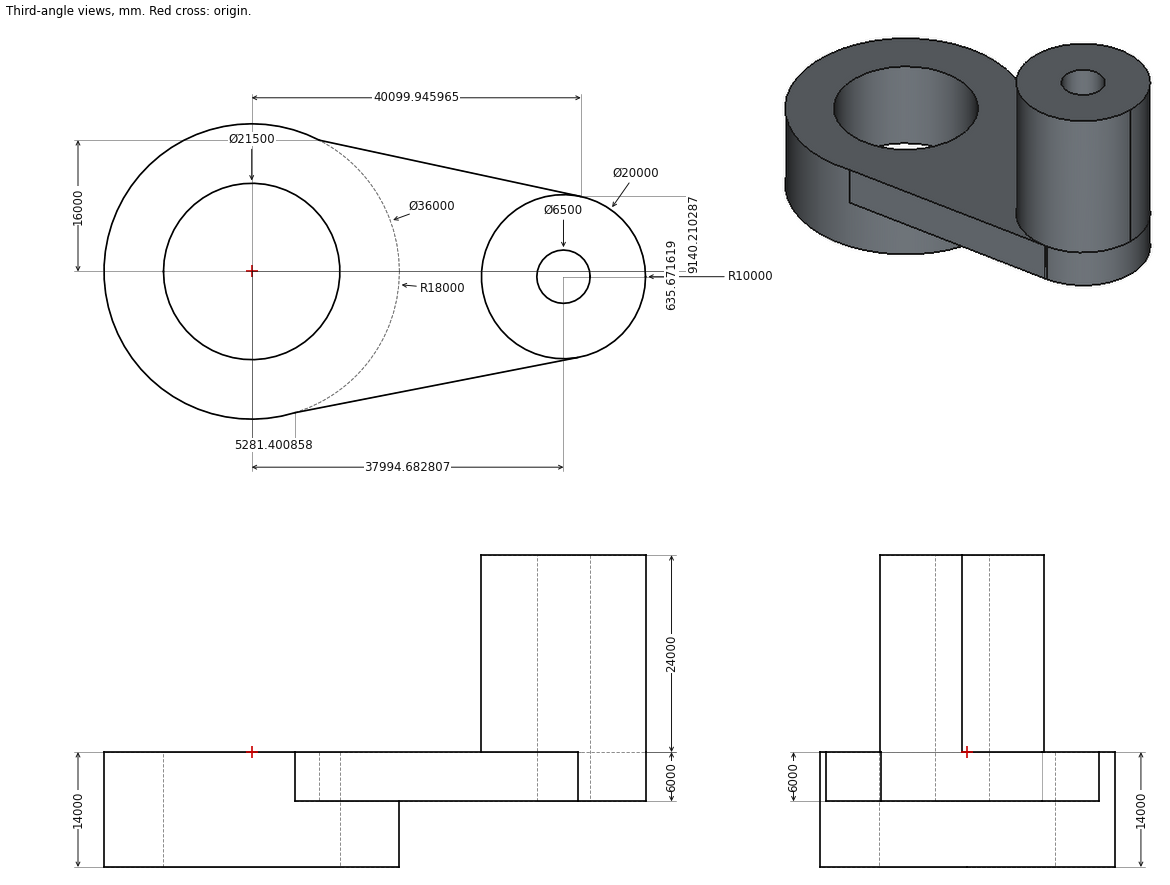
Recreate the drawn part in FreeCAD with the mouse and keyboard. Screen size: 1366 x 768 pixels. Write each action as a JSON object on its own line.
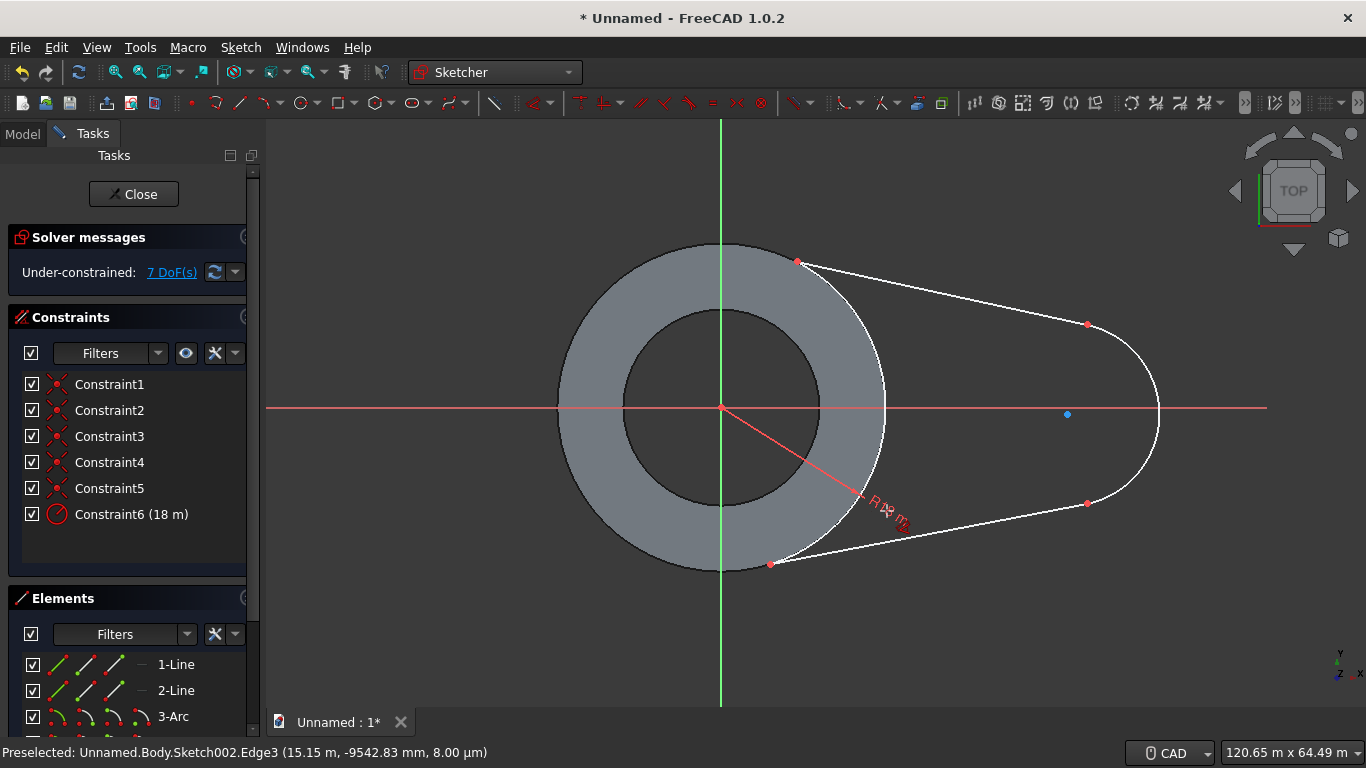
{"action": "left_click", "coordinate": [1146, 462]}
{"action": "left_click", "coordinate": [1173, 479]}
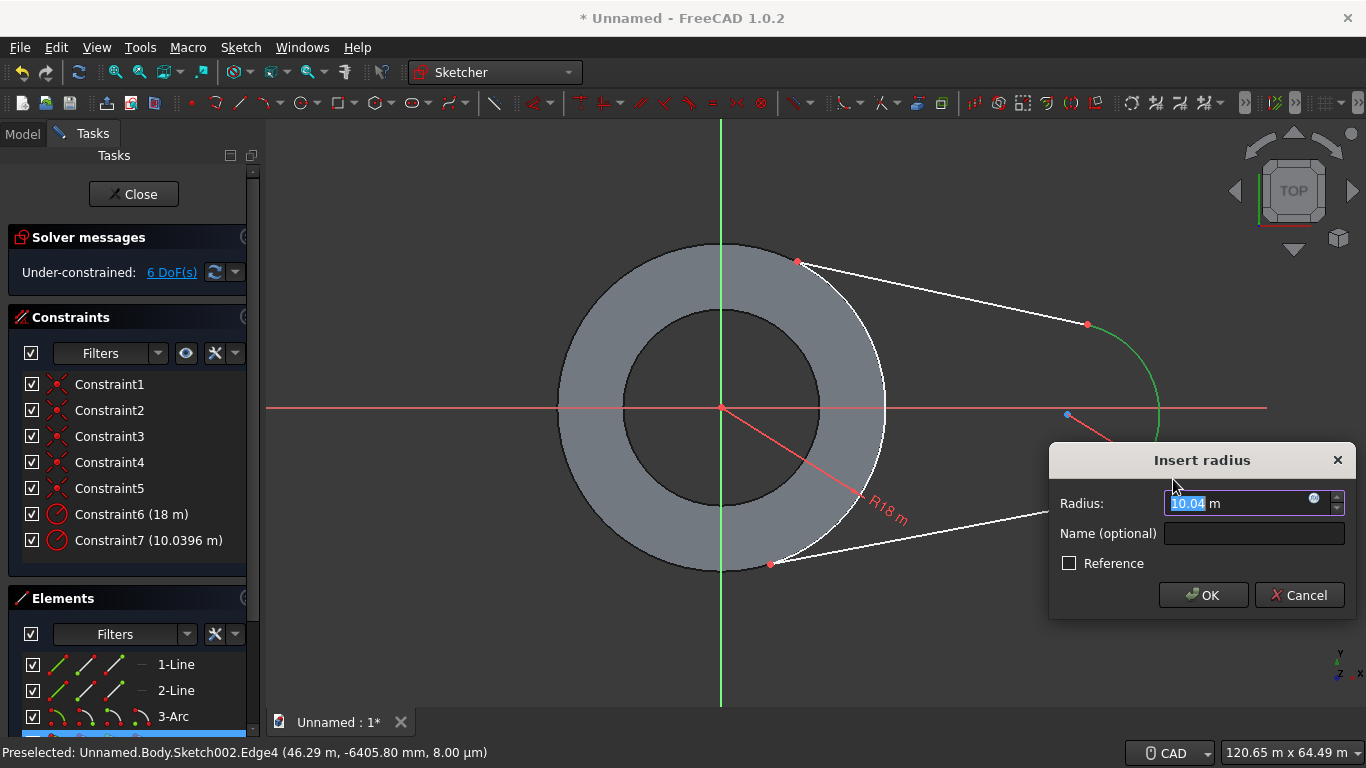
{"action": "key", "text": "ctrl+a"}
{"action": "type", "text": "10000 mm"}
{"action": "key", "text": "Return"}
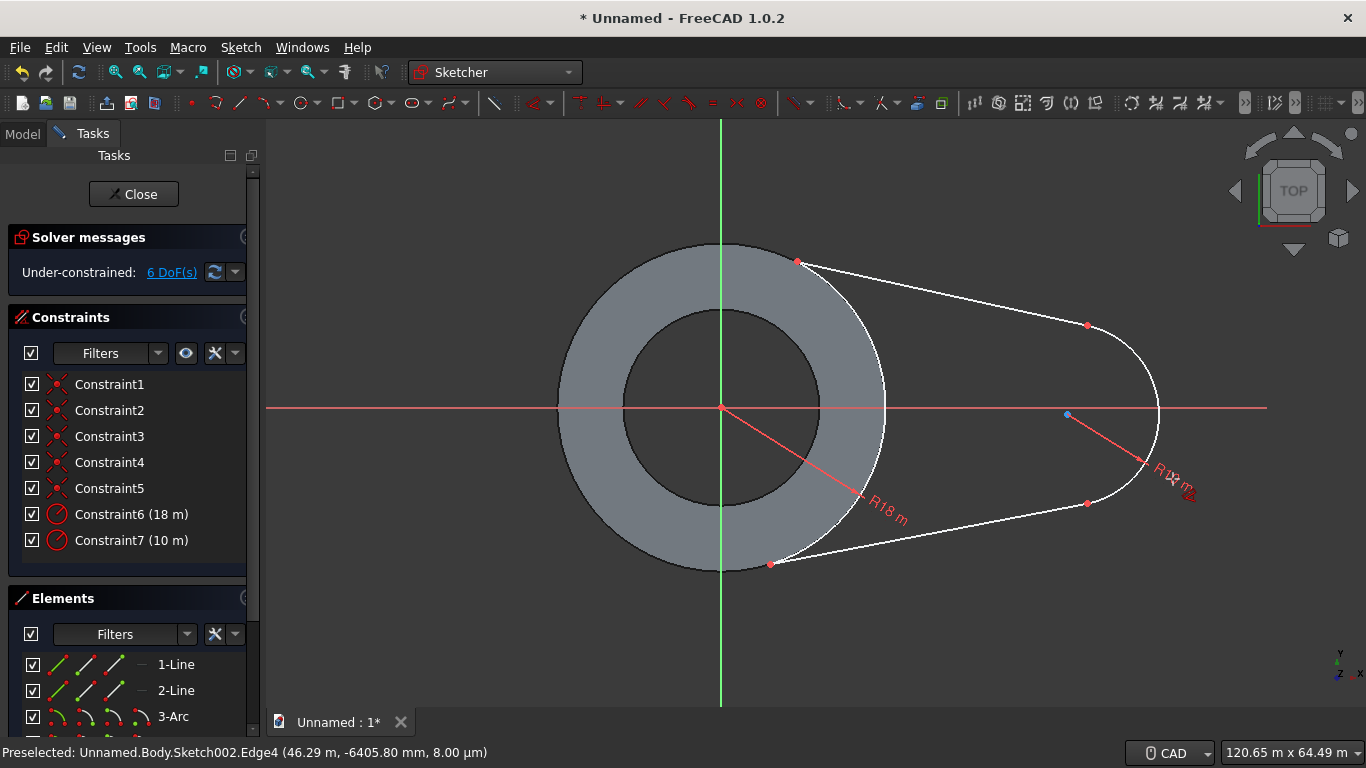
{"action": "left_click", "coordinate": [797, 262]}
{"action": "left_click", "coordinate": [687, 335]}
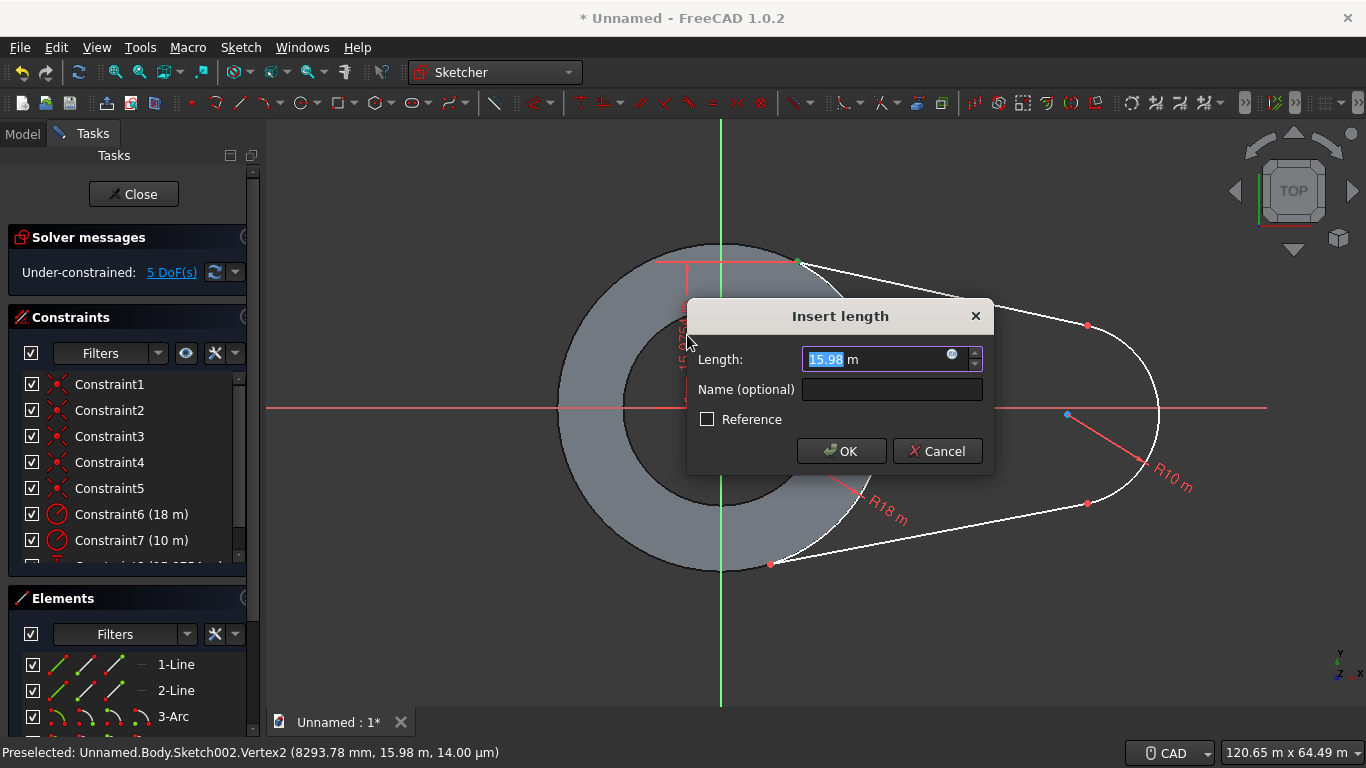
{"action": "key", "text": "ctrl+a"}
{"action": "type", "text": "16000 mm"}
{"action": "key", "text": "Return"}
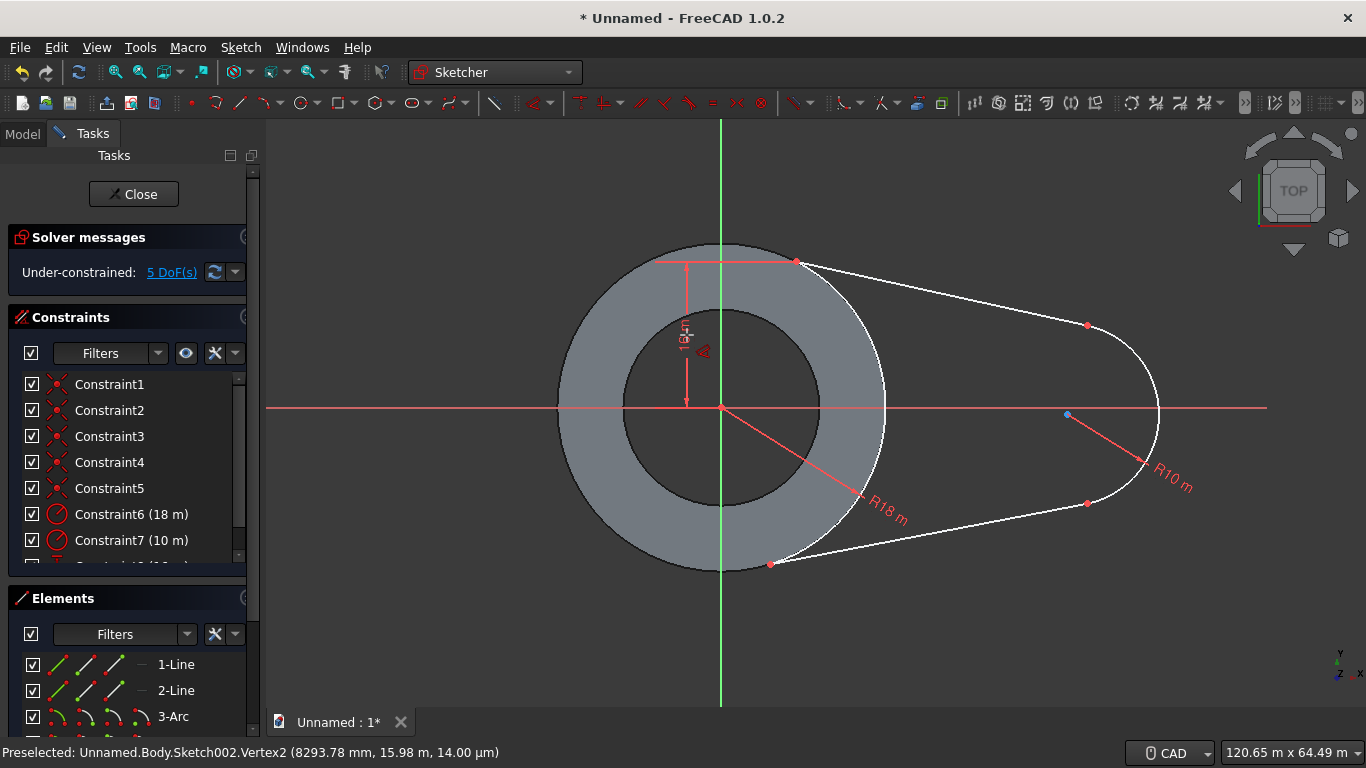
{"action": "scroll", "coordinate": [1068, 415], "scroll_direction": "up", "scroll_amount": 10}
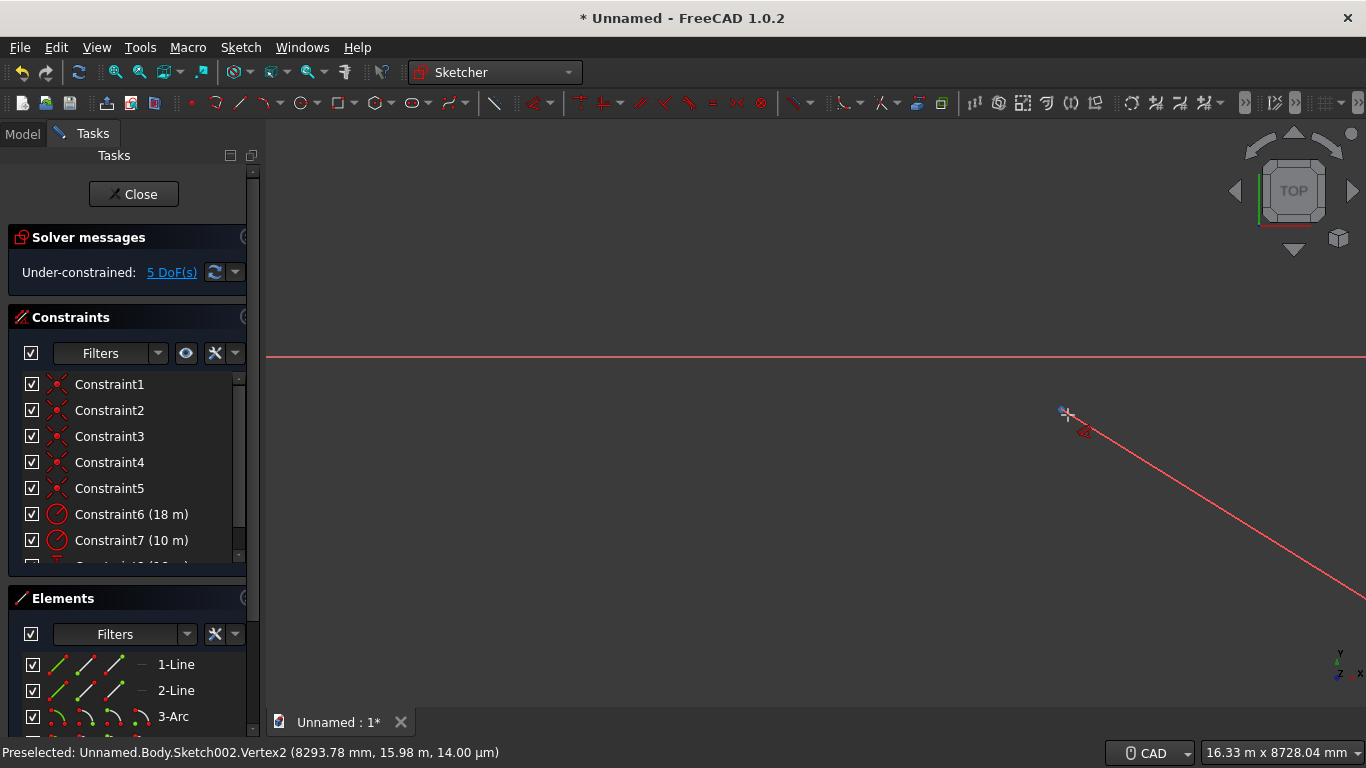
{"action": "left_click", "coordinate": [1062, 409]}
{"action": "left_click", "coordinate": [1096, 383]}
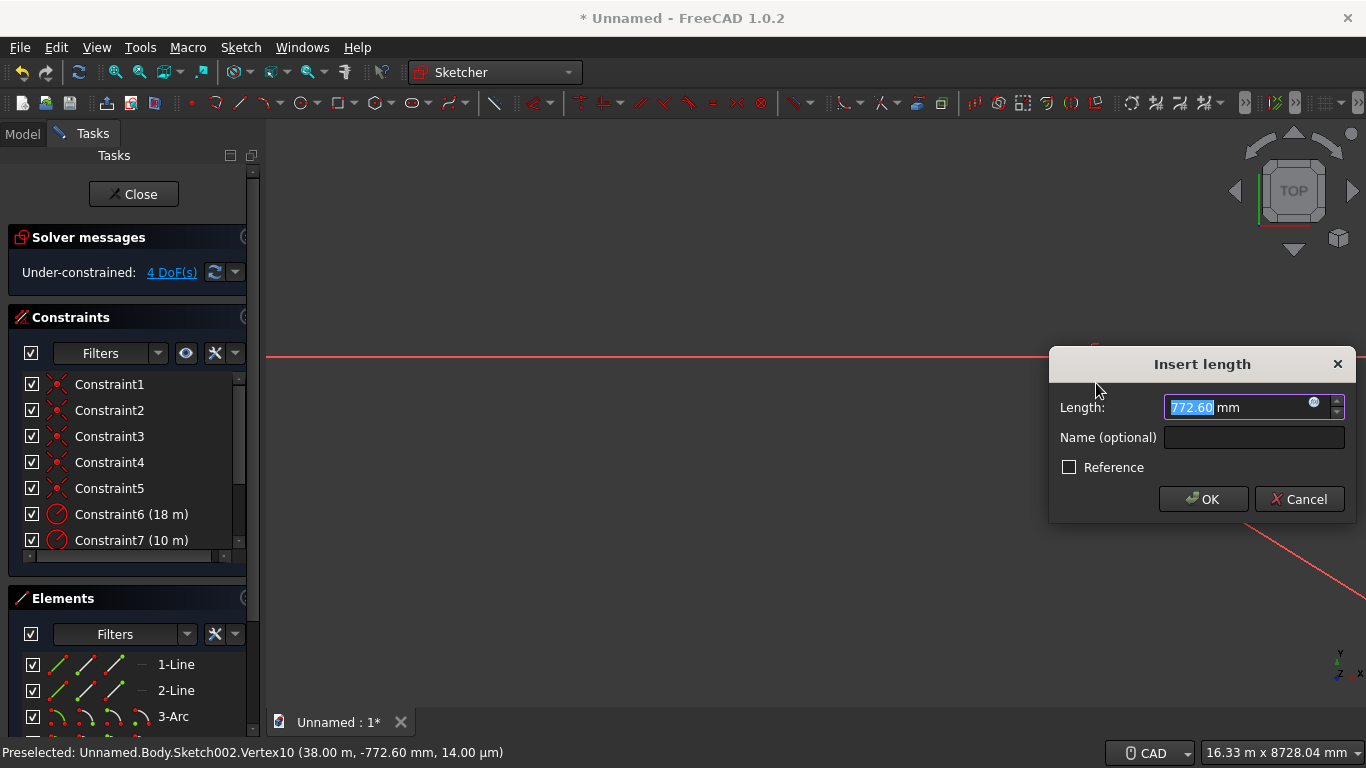
{"action": "type", "text": "635.671619"}
{"action": "key", "text": "Return"}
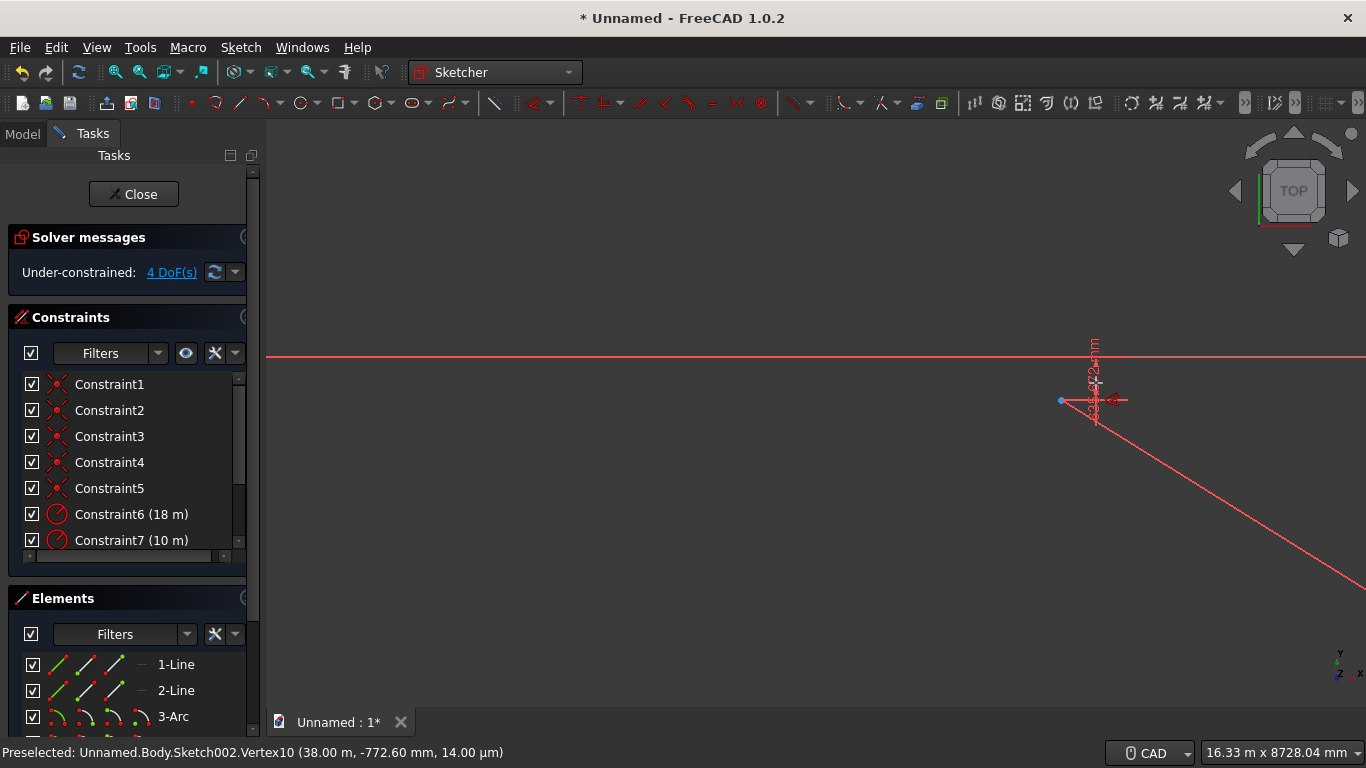
{"action": "scroll", "coordinate": [872, 416], "scroll_direction": "down", "scroll_amount": 9}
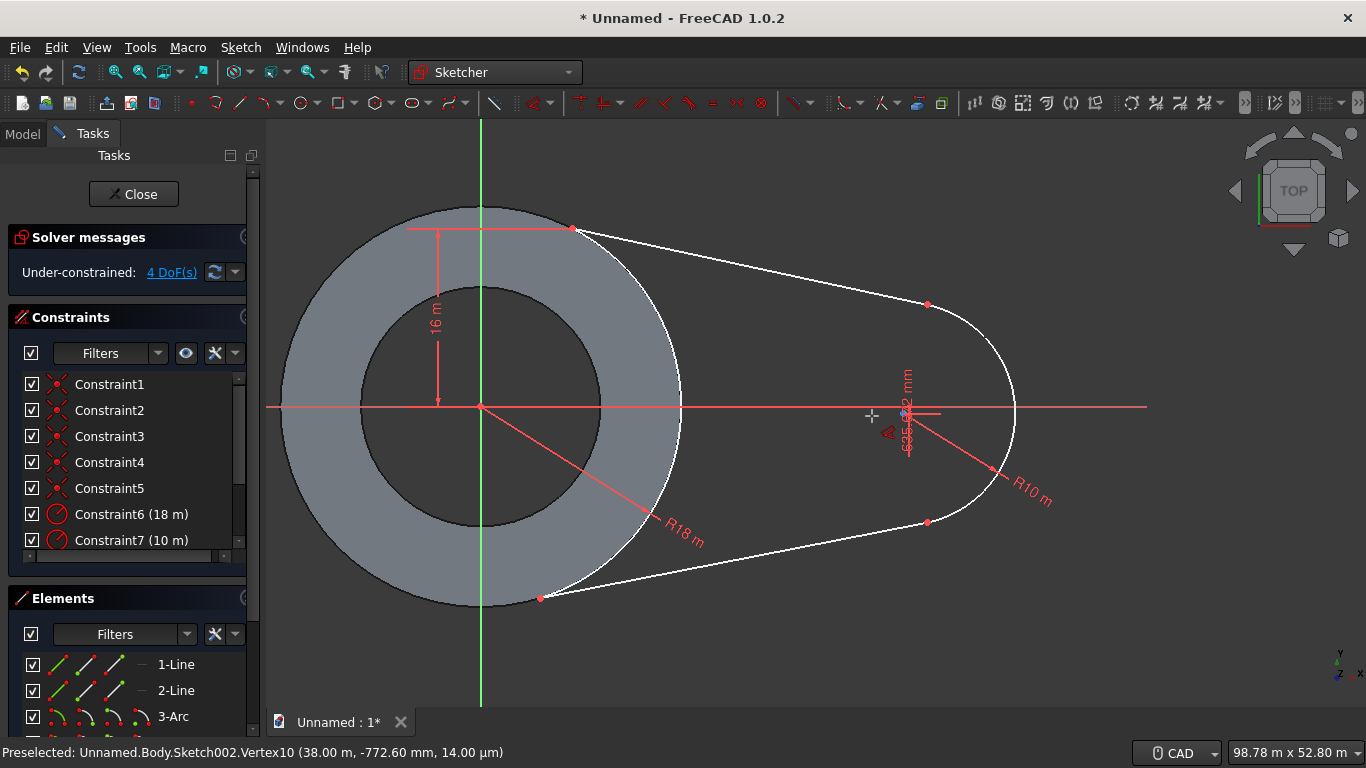
{"action": "left_click", "coordinate": [927, 305]}
{"action": "left_click", "coordinate": [447, 356]}